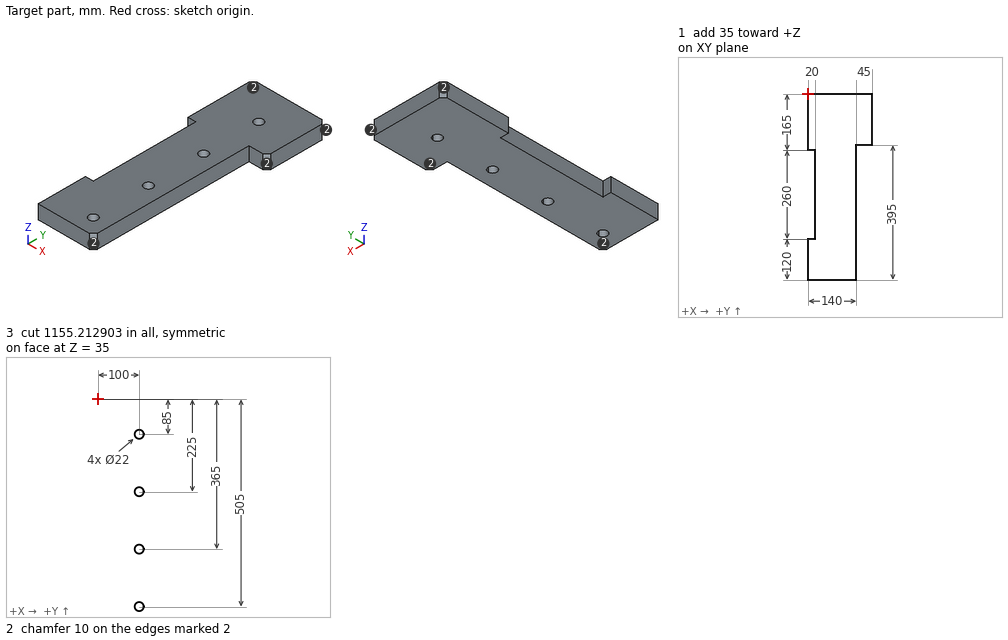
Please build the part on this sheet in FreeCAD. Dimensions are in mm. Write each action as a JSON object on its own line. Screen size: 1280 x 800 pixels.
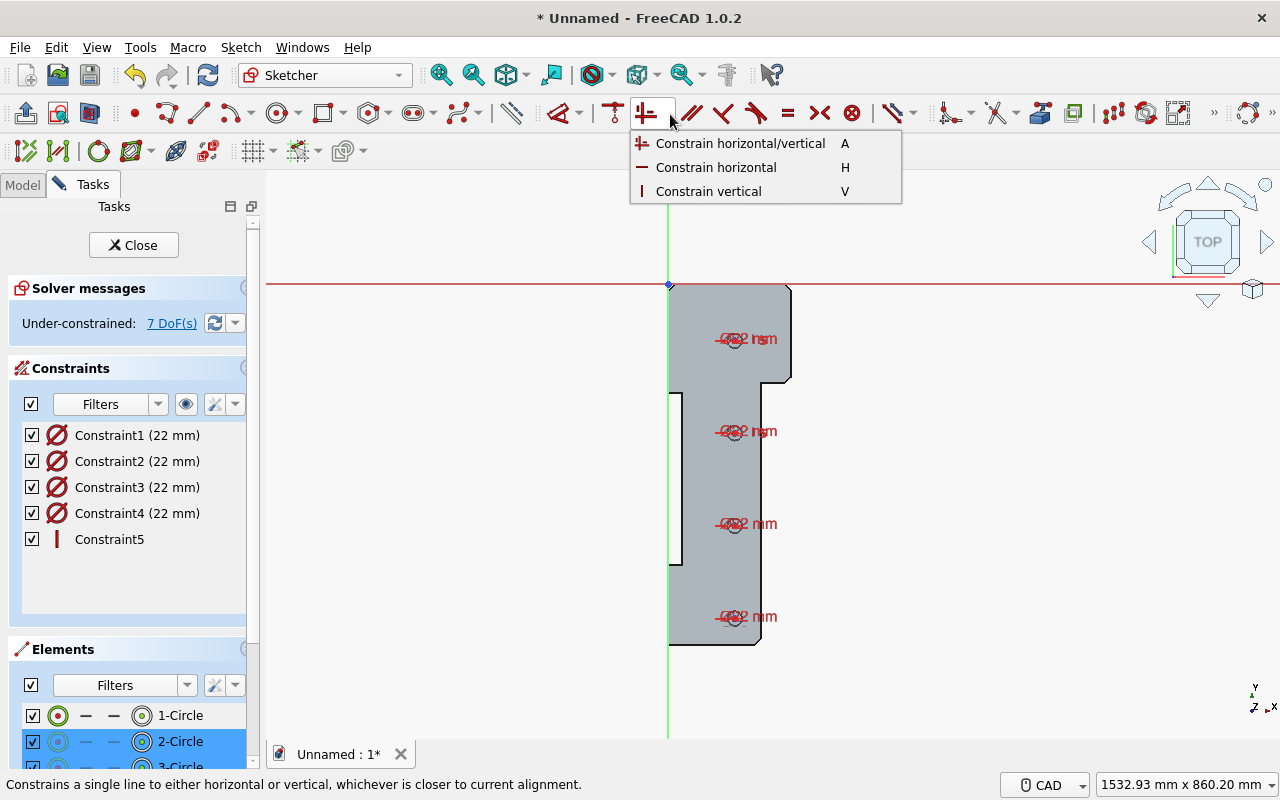
{"action": "left_click", "coordinate": [766, 191]}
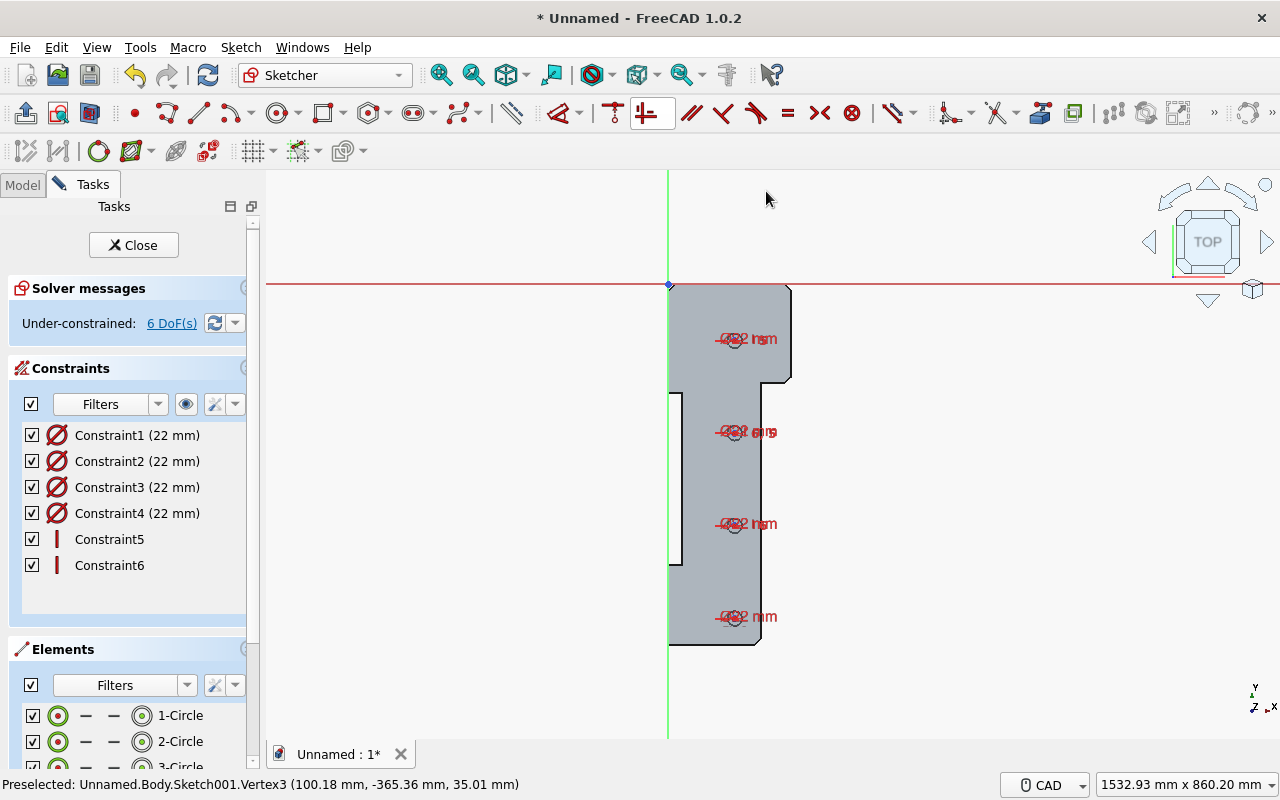
{"action": "left_click", "coordinate": [735, 526]}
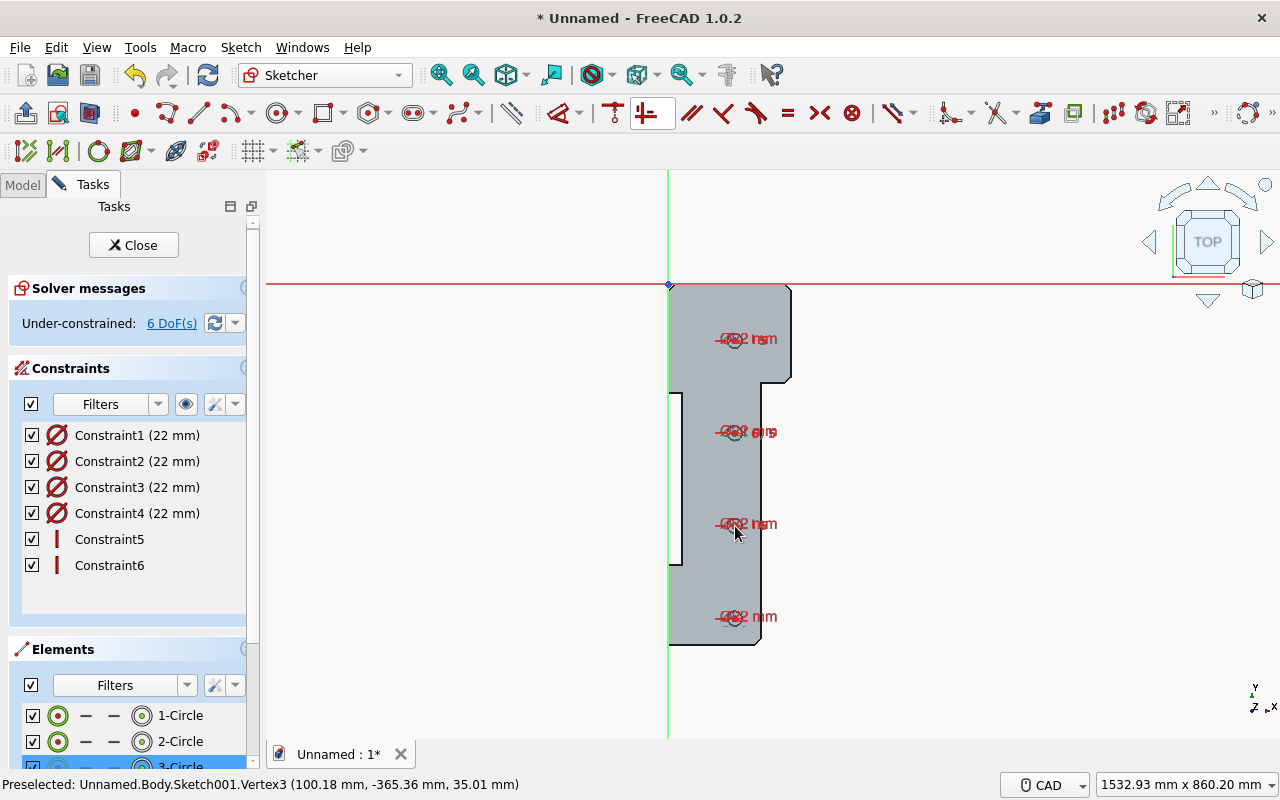
{"action": "left_click", "coordinate": [735, 619]}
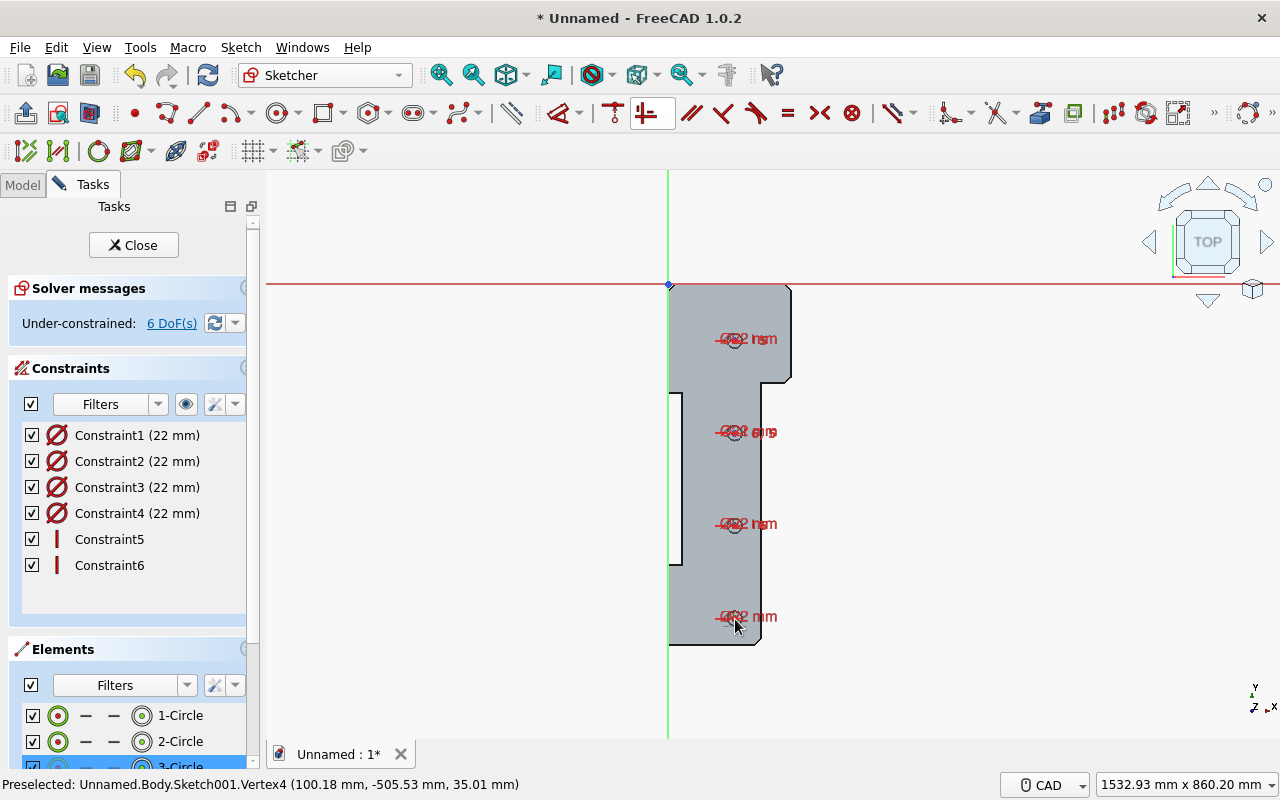
{"action": "left_click", "coordinate": [670, 114]}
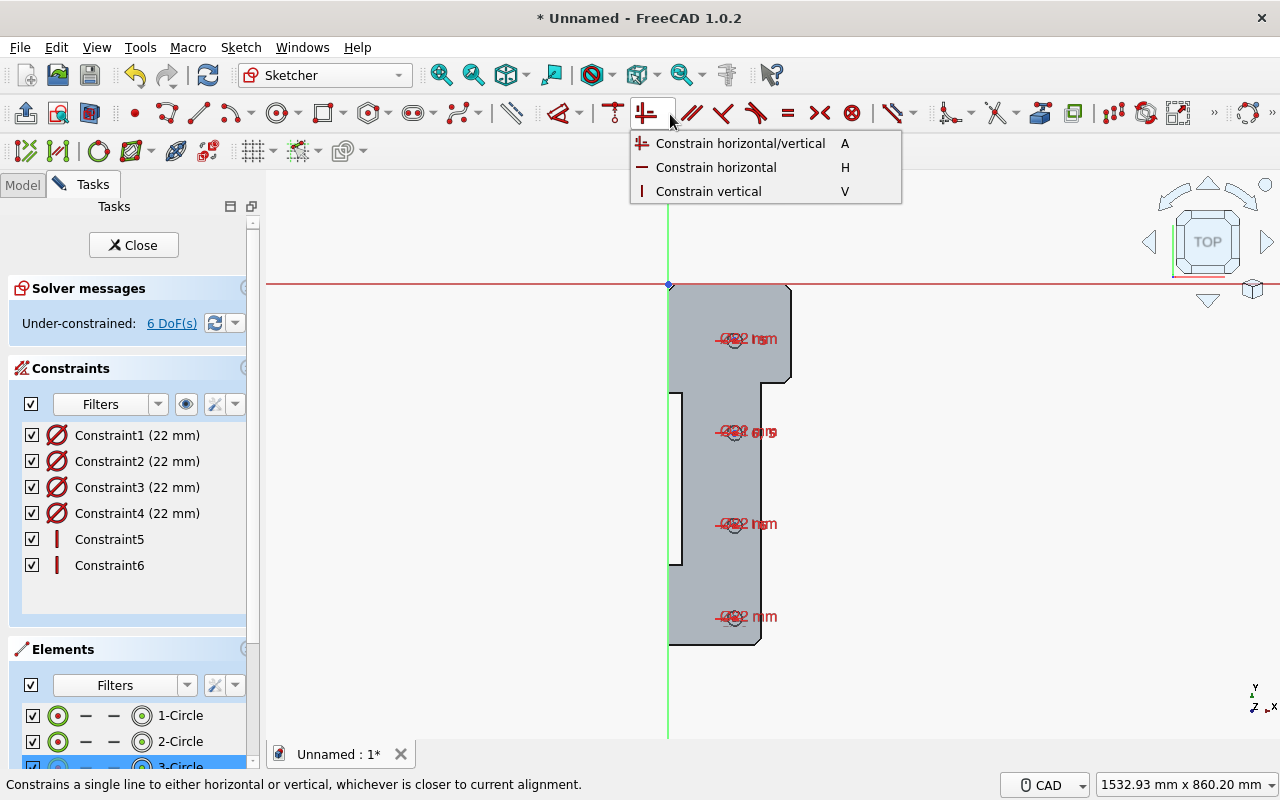
{"action": "left_click", "coordinate": [766, 191]}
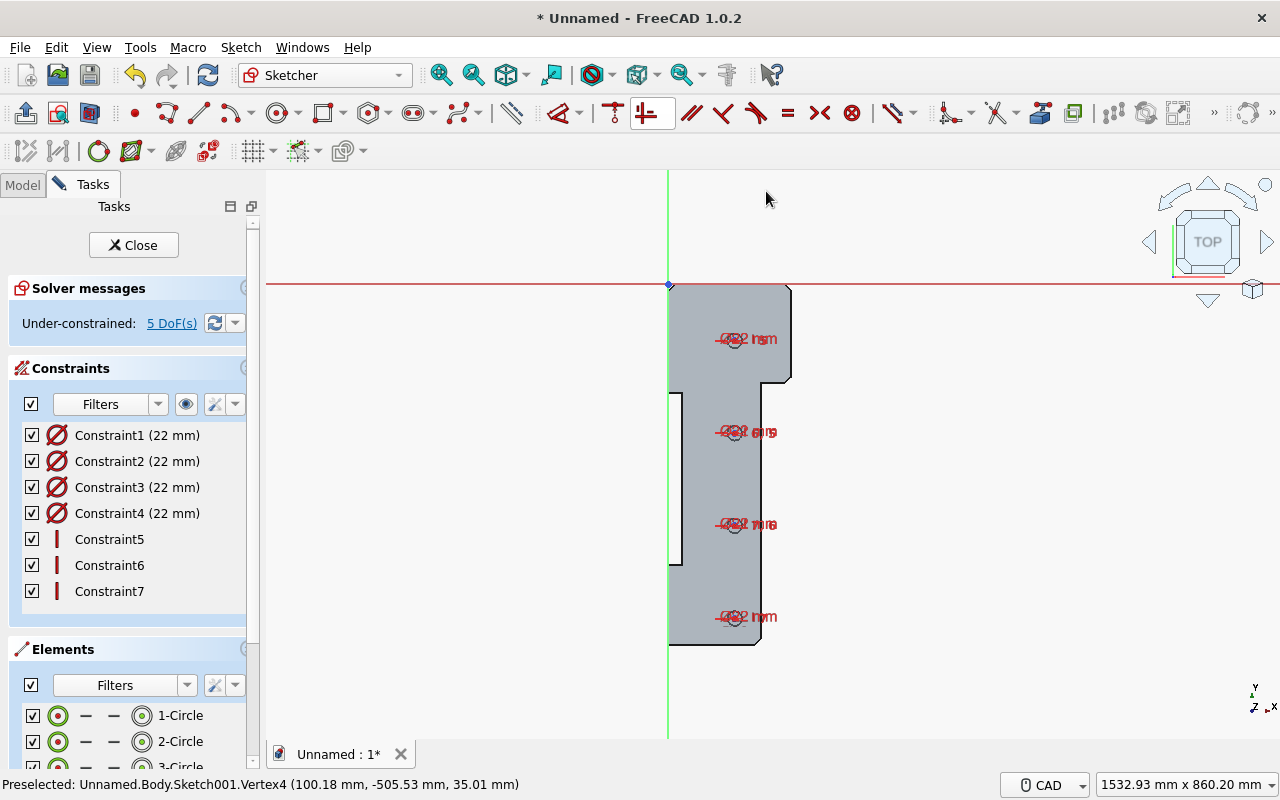
{"action": "left_click", "coordinate": [558, 114]}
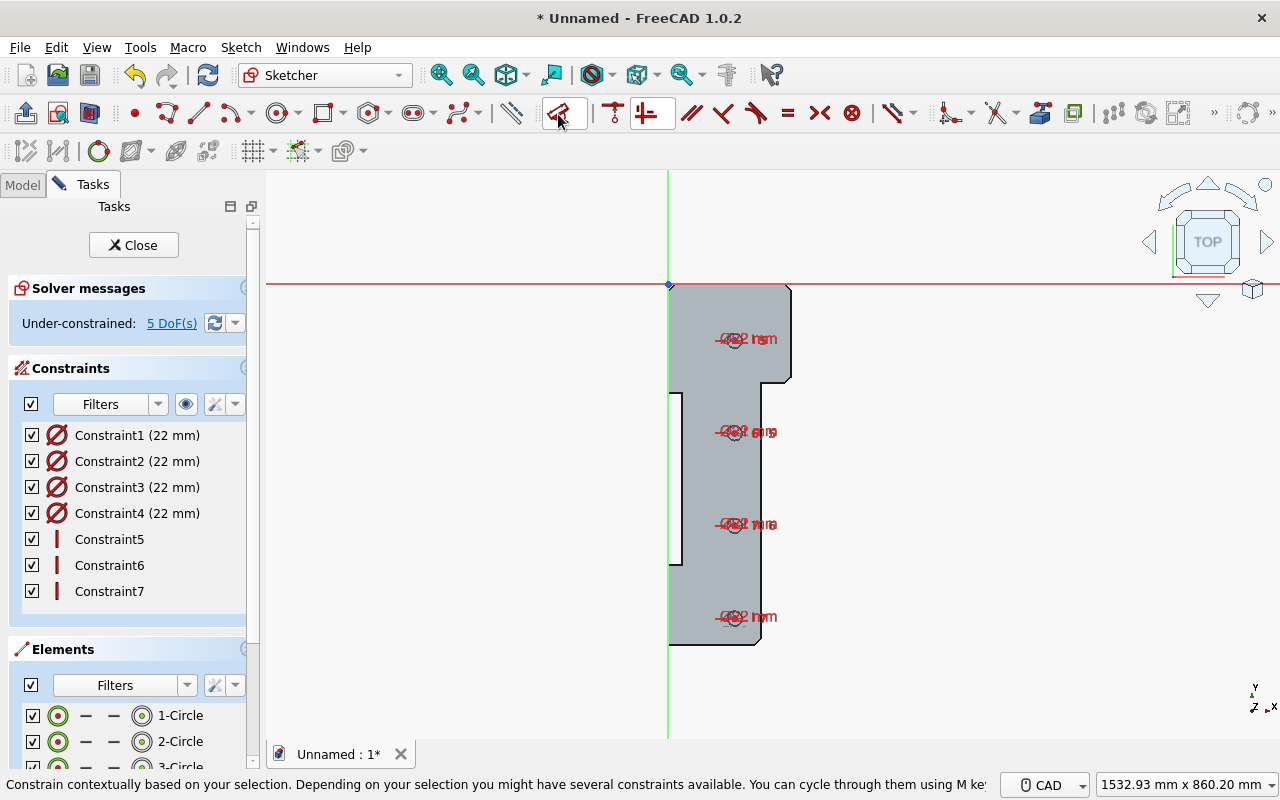
{"action": "left_click", "coordinate": [735, 341]}
{"action": "left_click", "coordinate": [634, 312]}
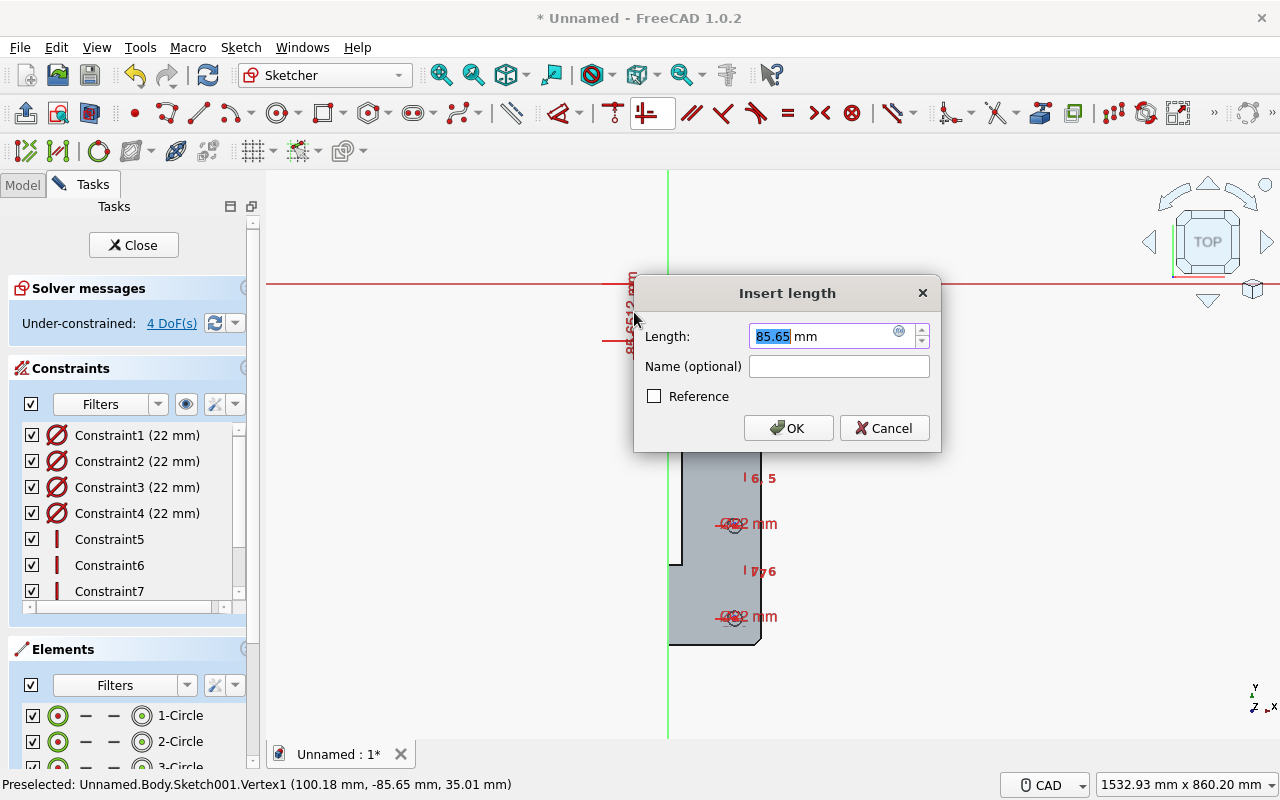
{"action": "type", "text": "85"}
{"action": "key", "text": "Return"}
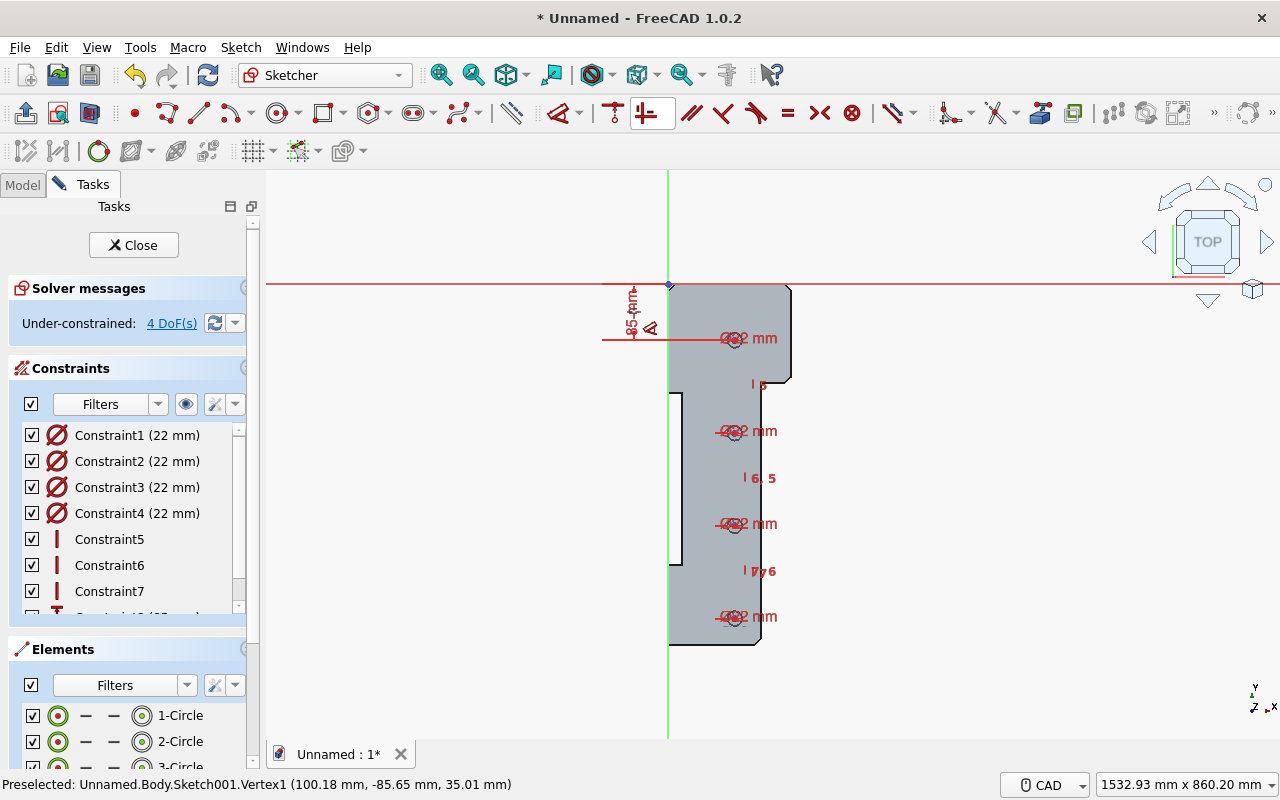
{"action": "left_click", "coordinate": [735, 340]}
{"action": "left_click", "coordinate": [702, 250]}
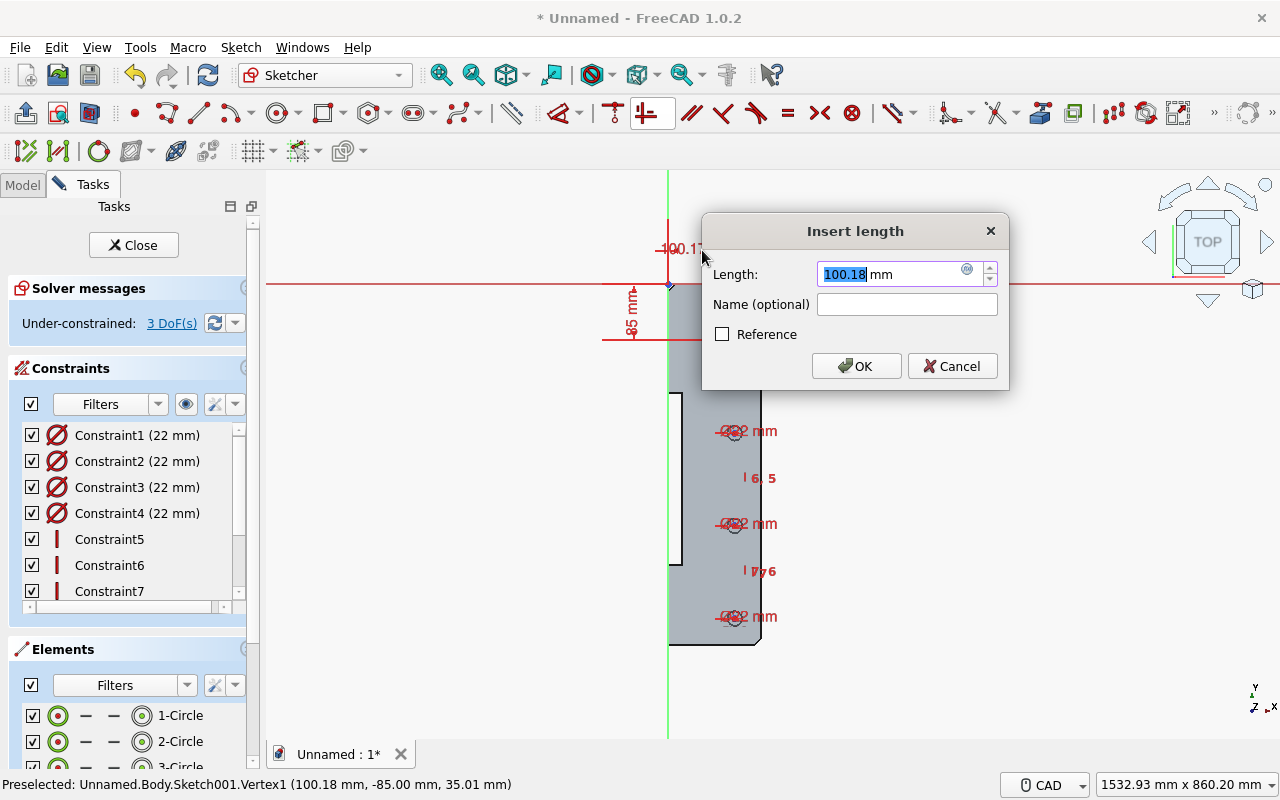
{"action": "type", "text": "100"}
{"action": "key", "text": "Return"}